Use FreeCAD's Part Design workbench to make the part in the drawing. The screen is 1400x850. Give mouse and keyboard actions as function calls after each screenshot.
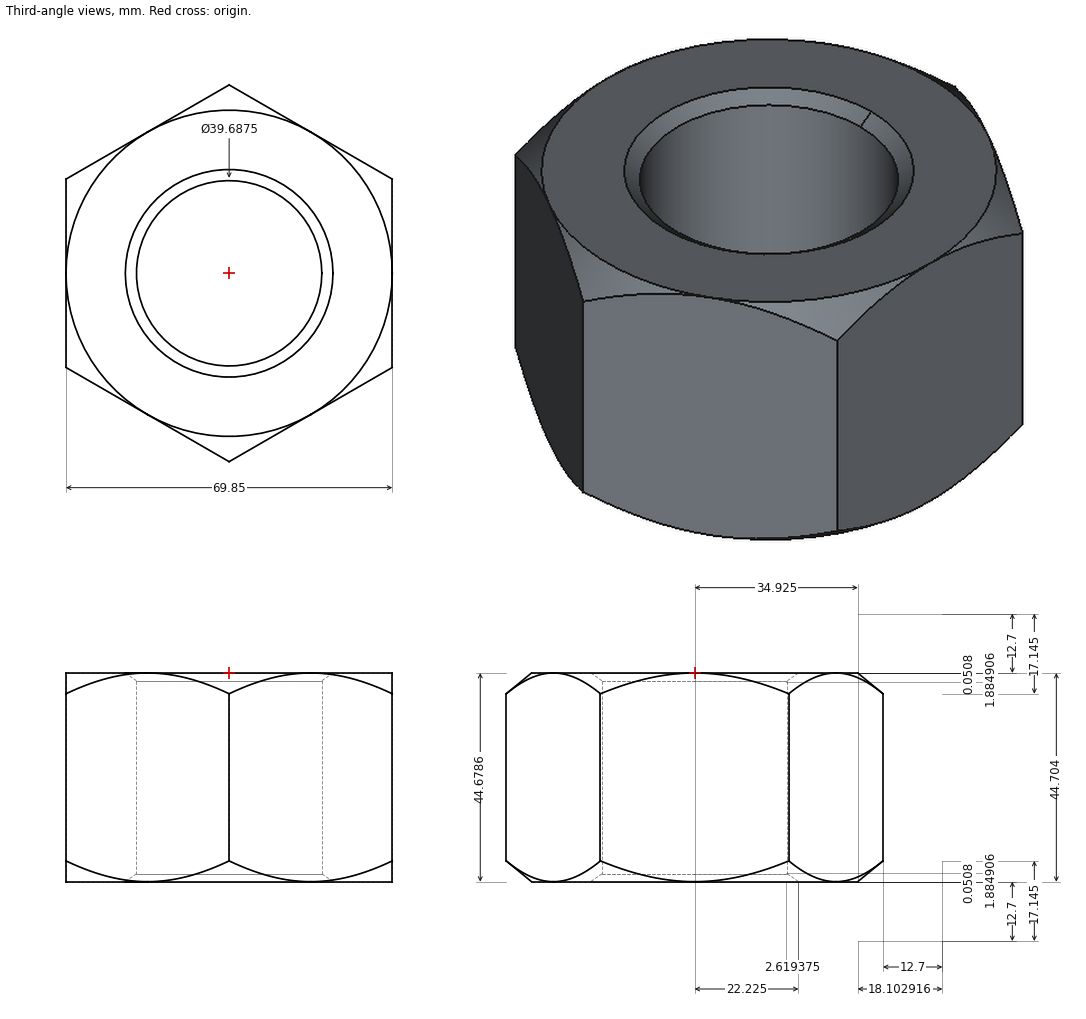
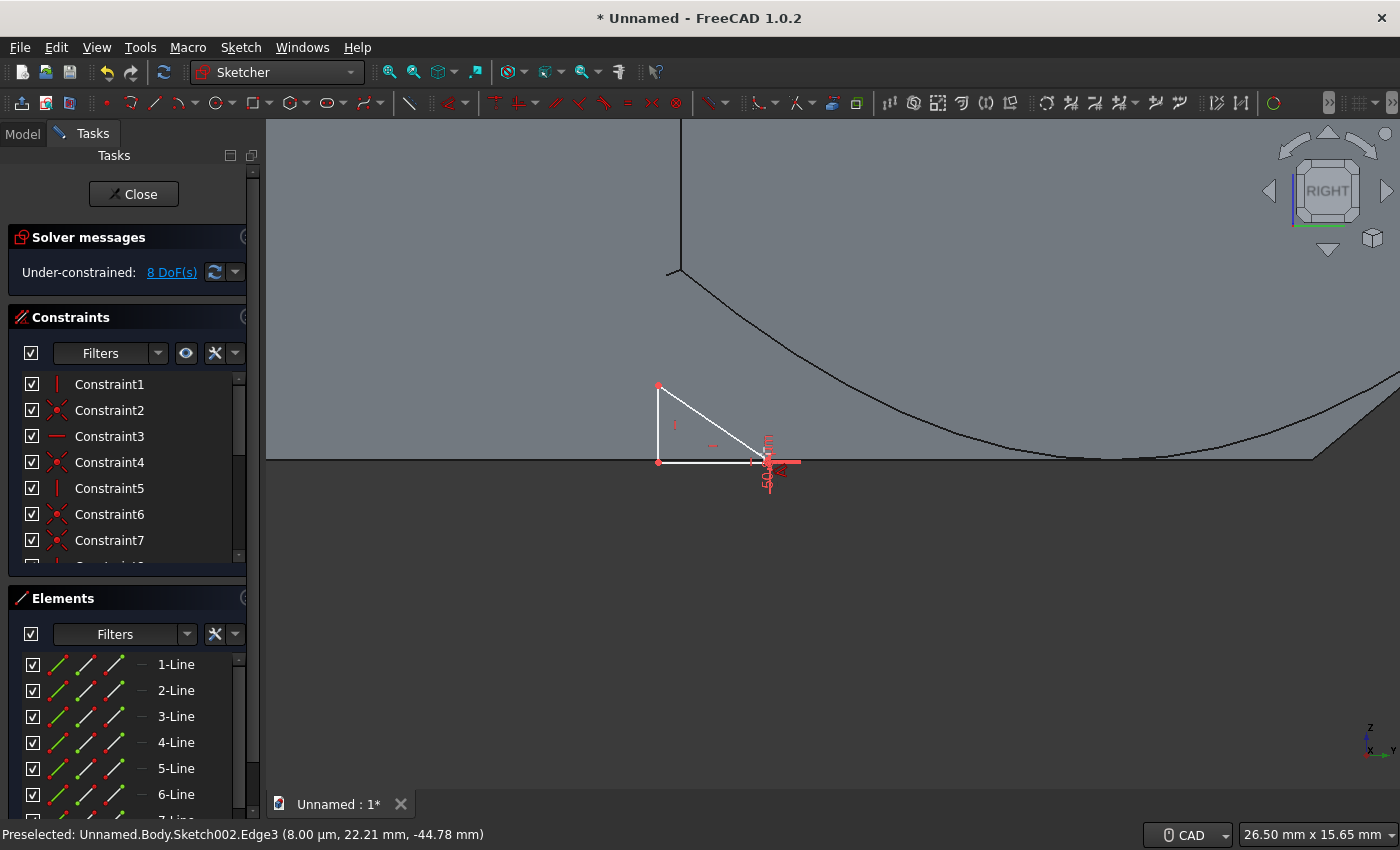
scroll(919, 761, down, 7)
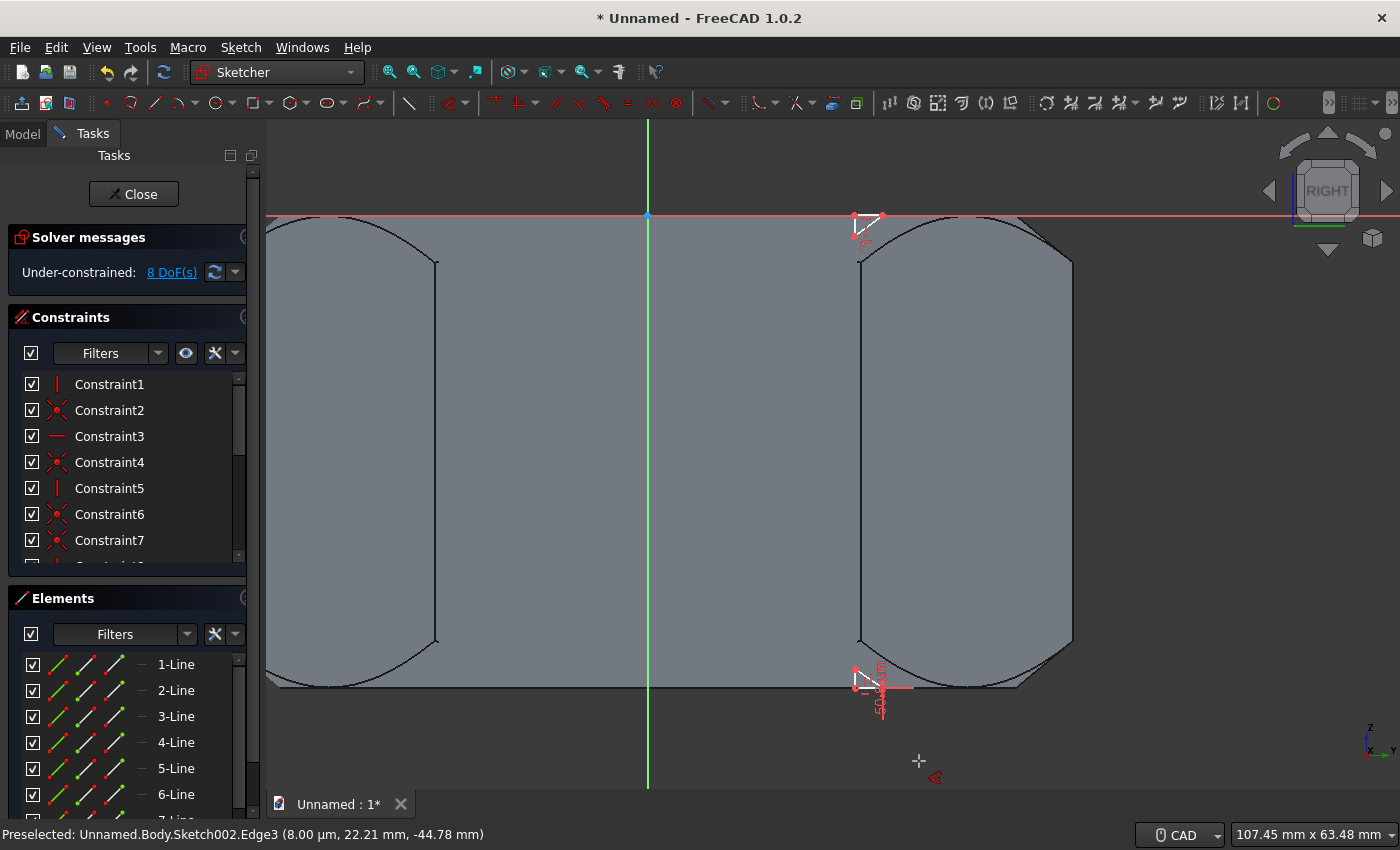
scroll(882, 216, up, 22)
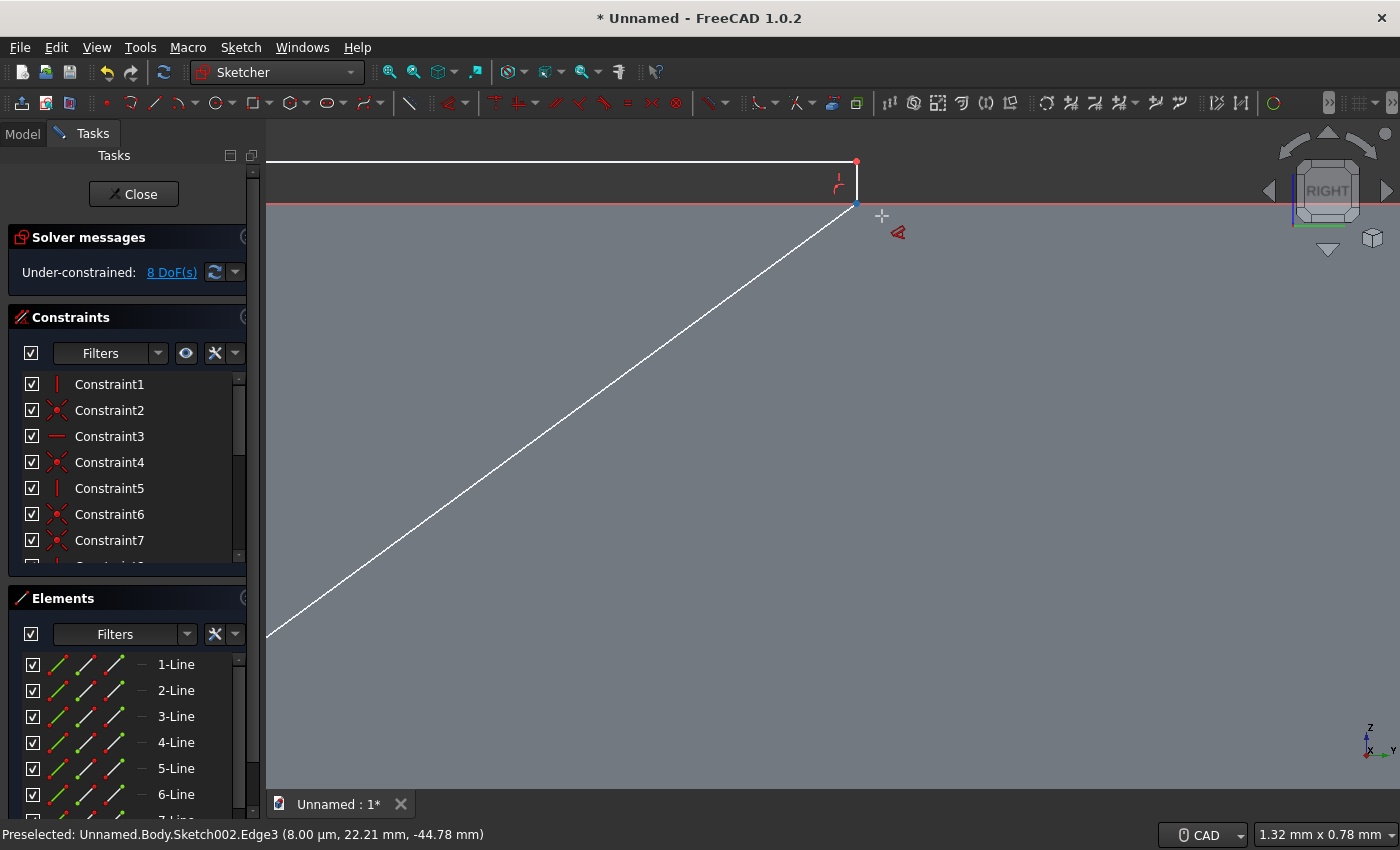
click(857, 191)
click(891, 183)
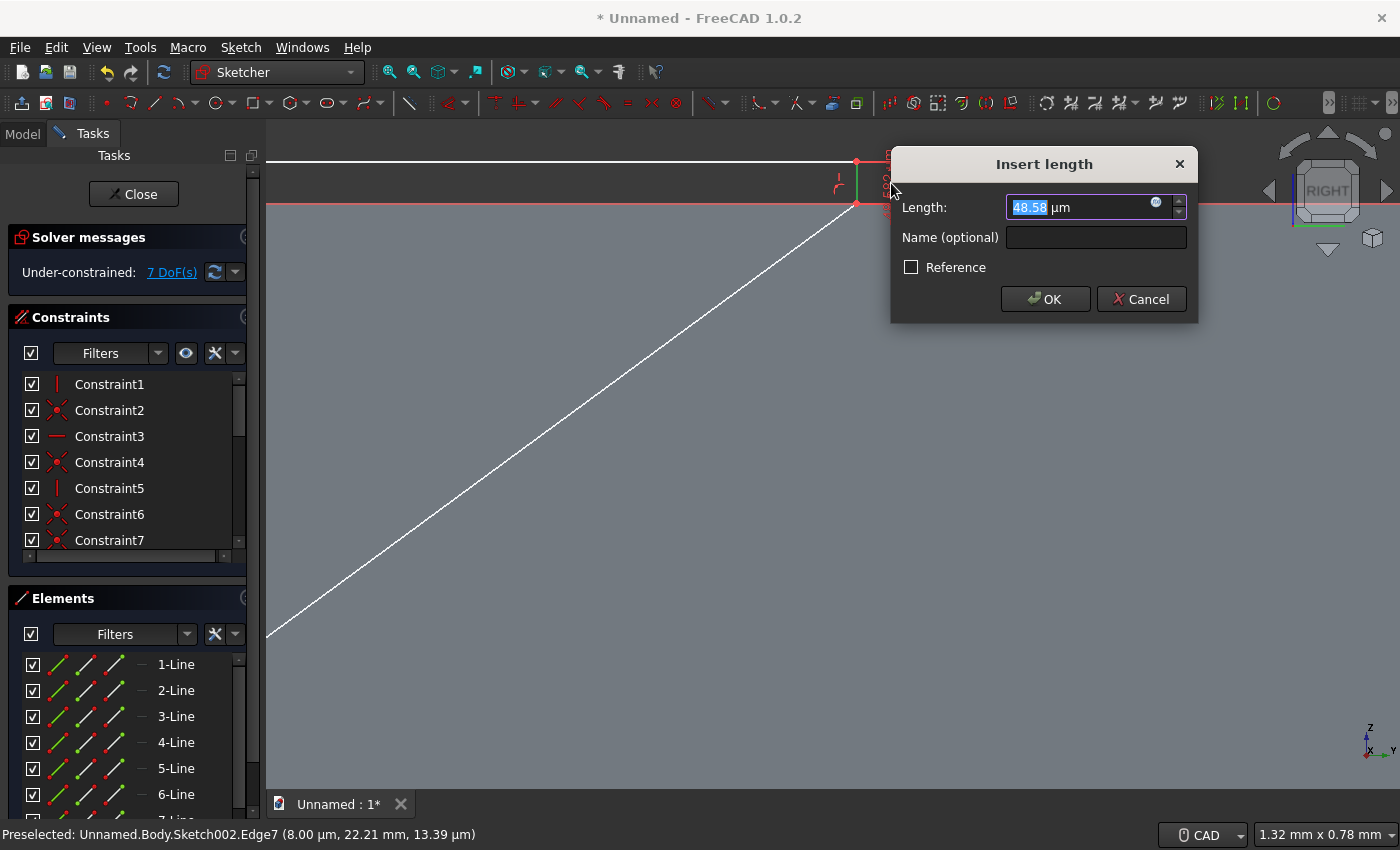
key(ctrl+a)
text(0.0508 mm)
key(Return)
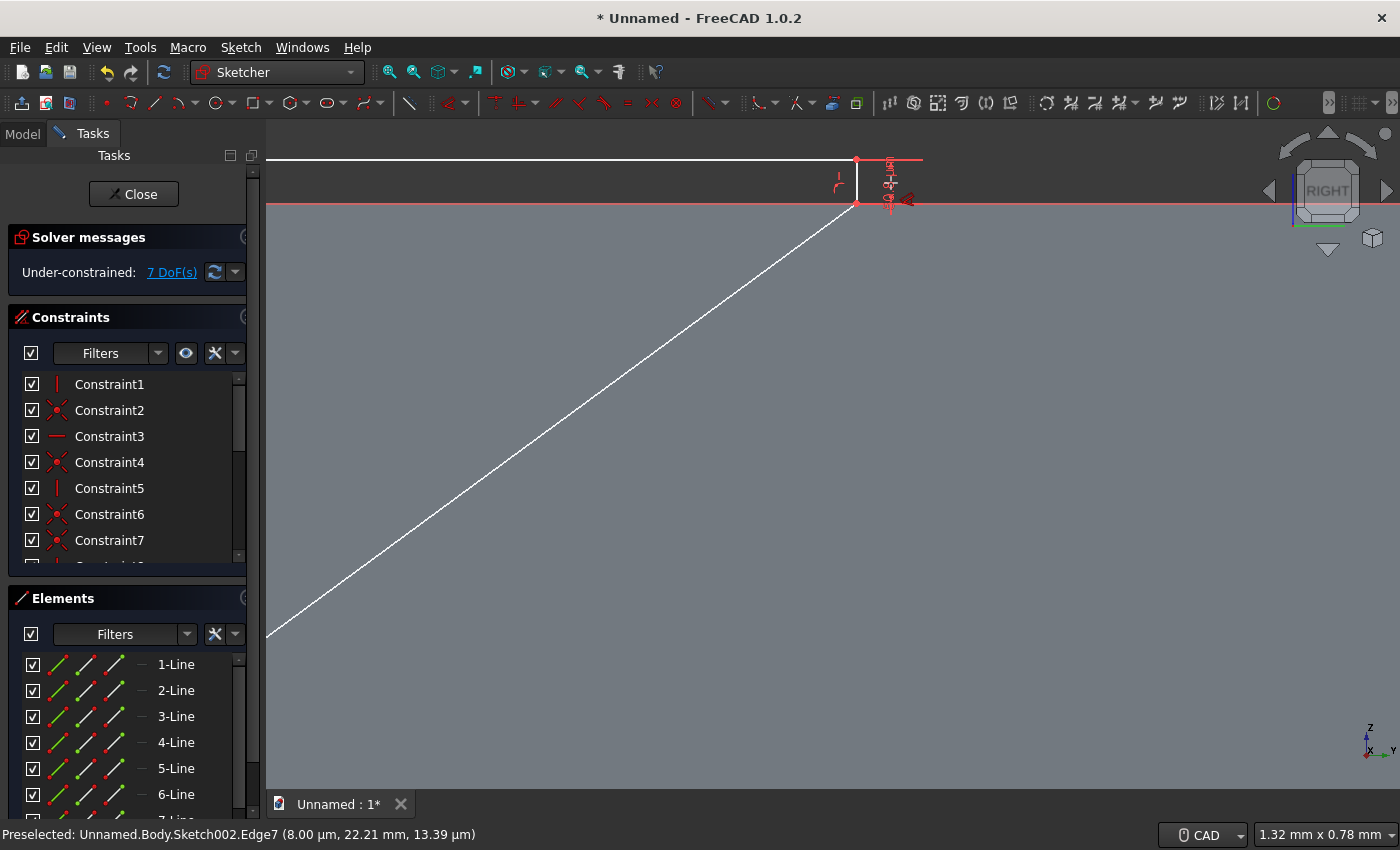
scroll(764, 454, down, 15)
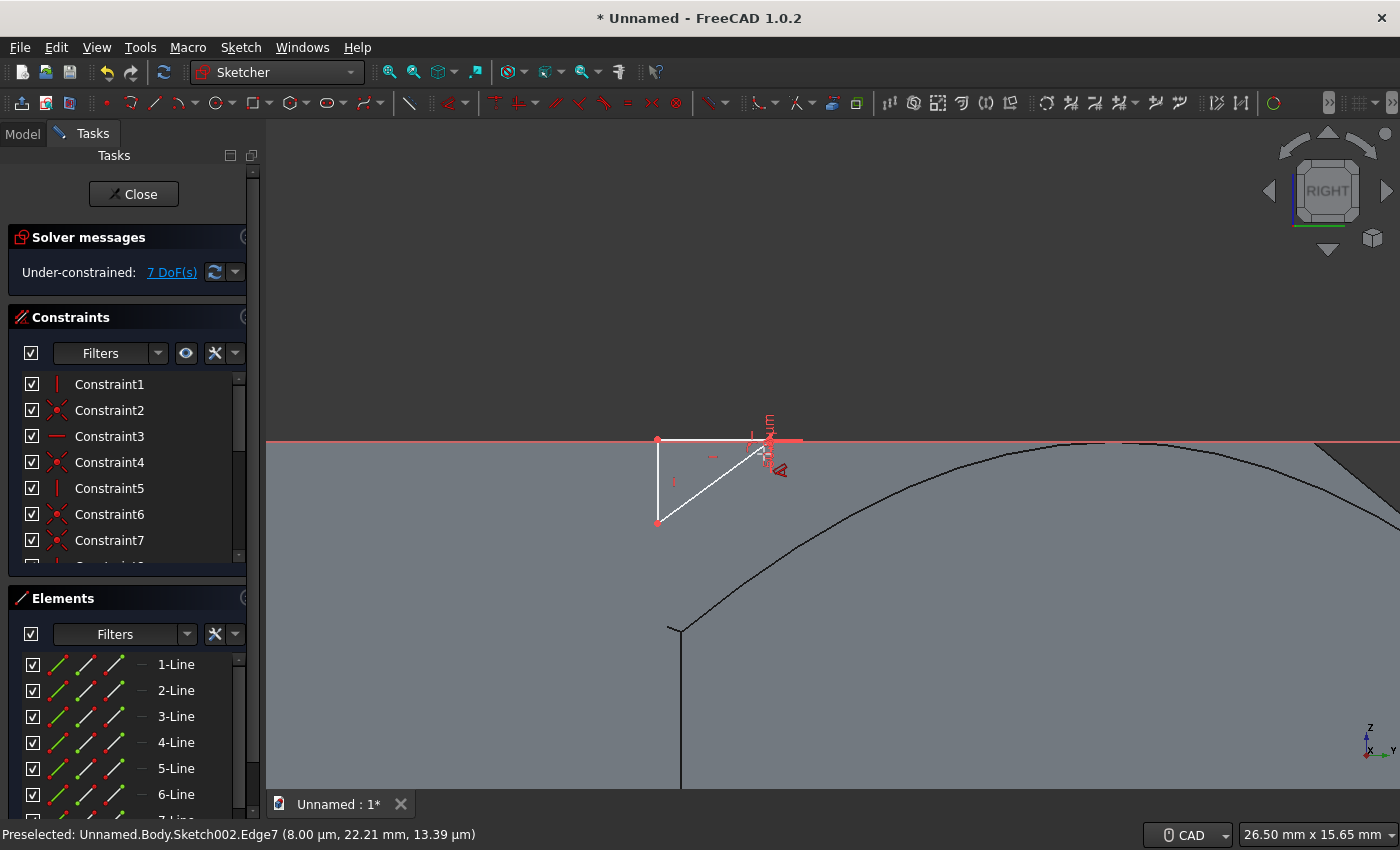
scroll(918, 147, down, 7)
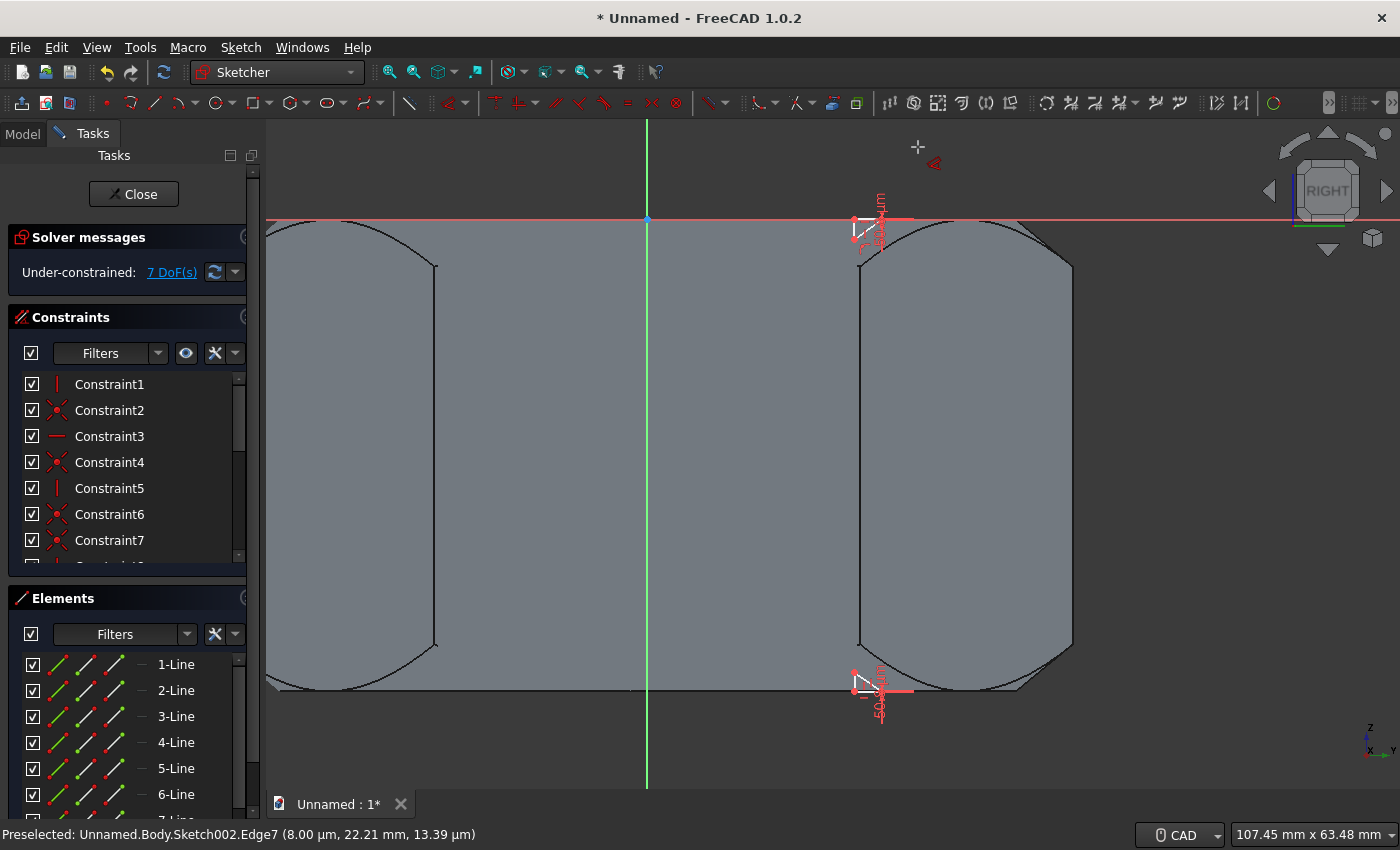
click(855, 692)
click(613, 456)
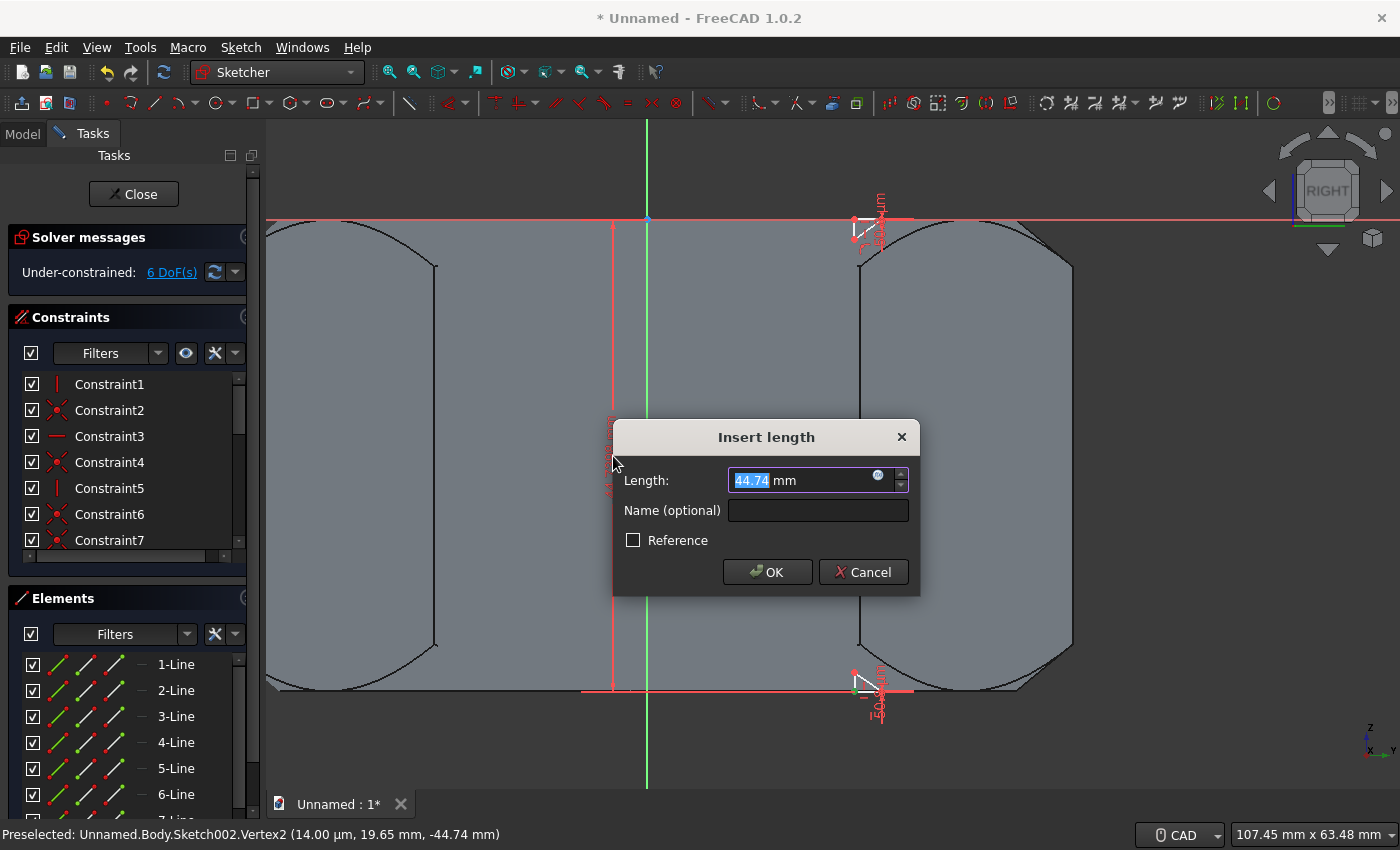
text(44.704)
key(Return)